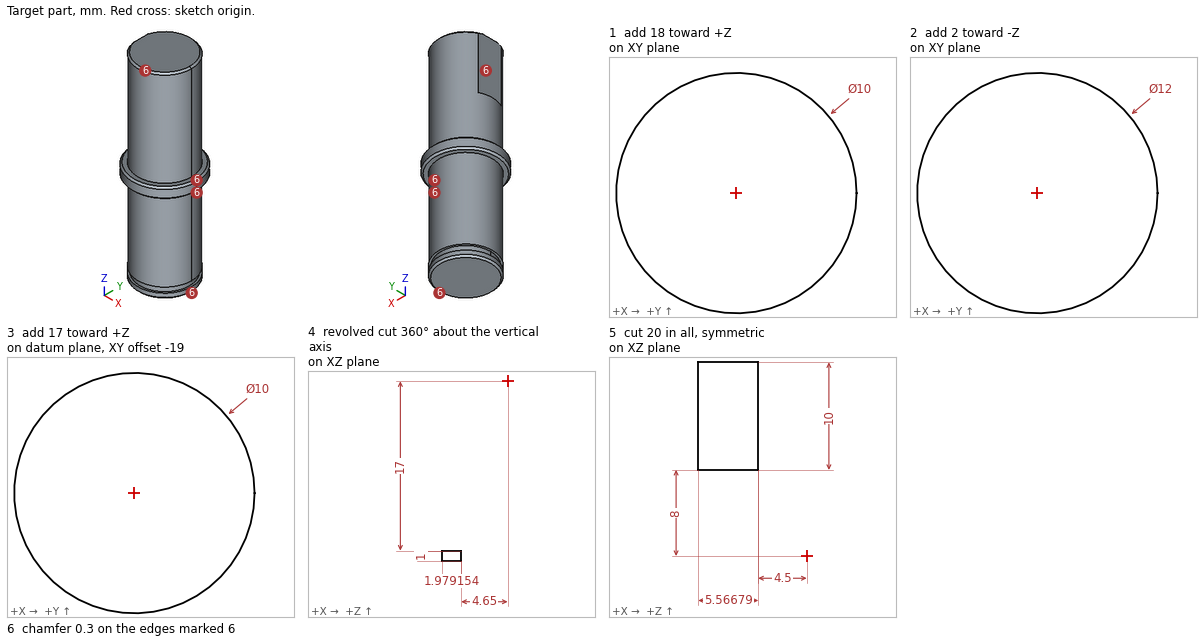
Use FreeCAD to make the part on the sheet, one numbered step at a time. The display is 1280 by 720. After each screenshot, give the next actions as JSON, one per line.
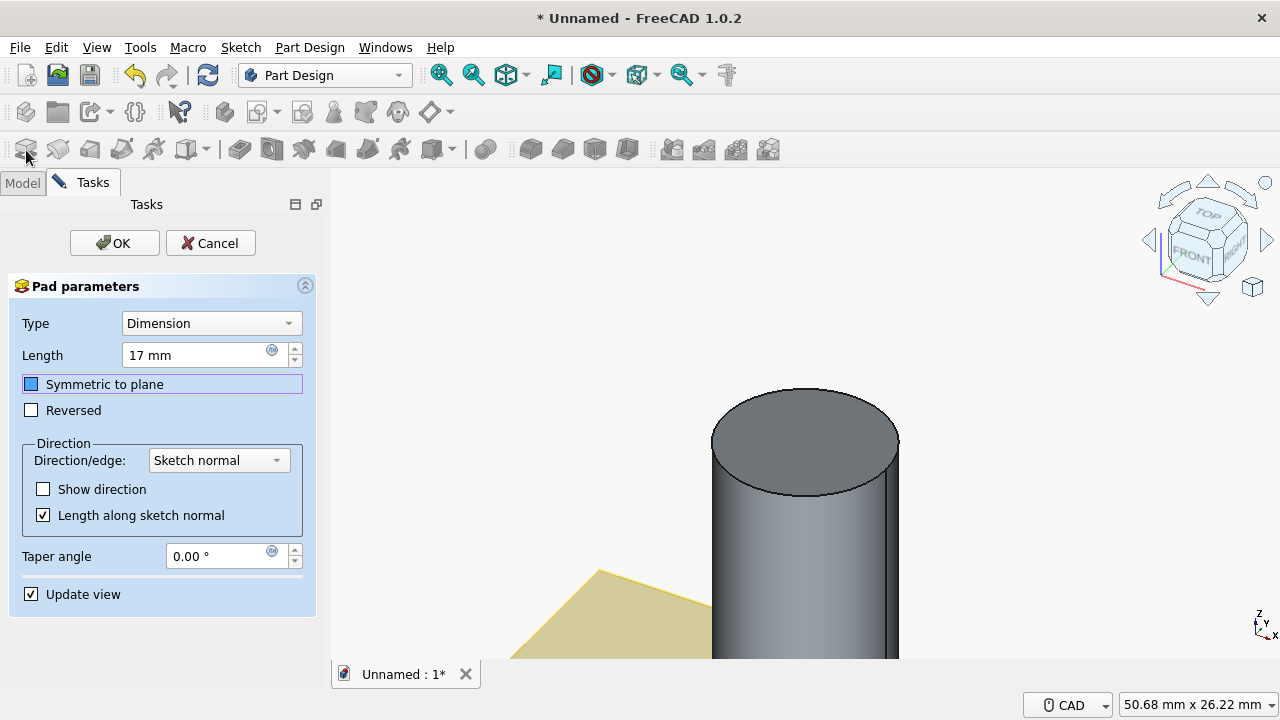
{"action": "left_click", "coordinate": [115, 243]}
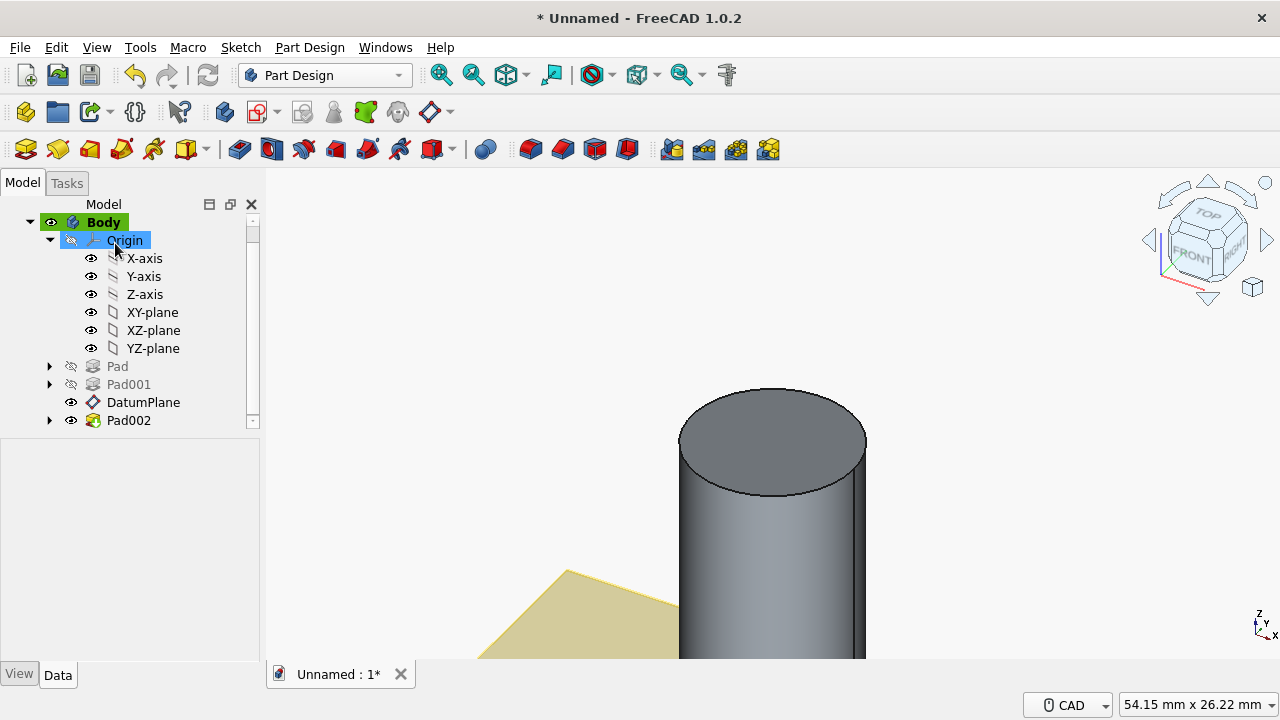
{"action": "left_click", "coordinate": [116, 402]}
{"action": "key", "text": "space"}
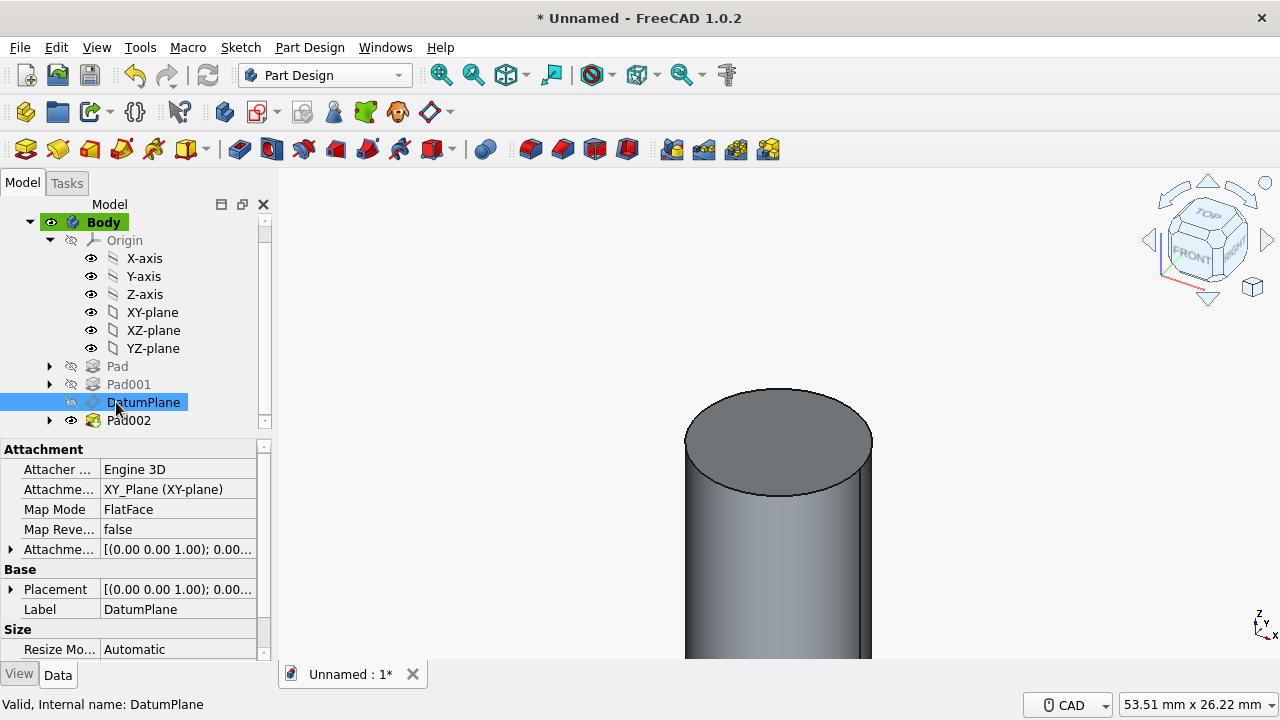
{"action": "left_click", "coordinate": [442, 76]}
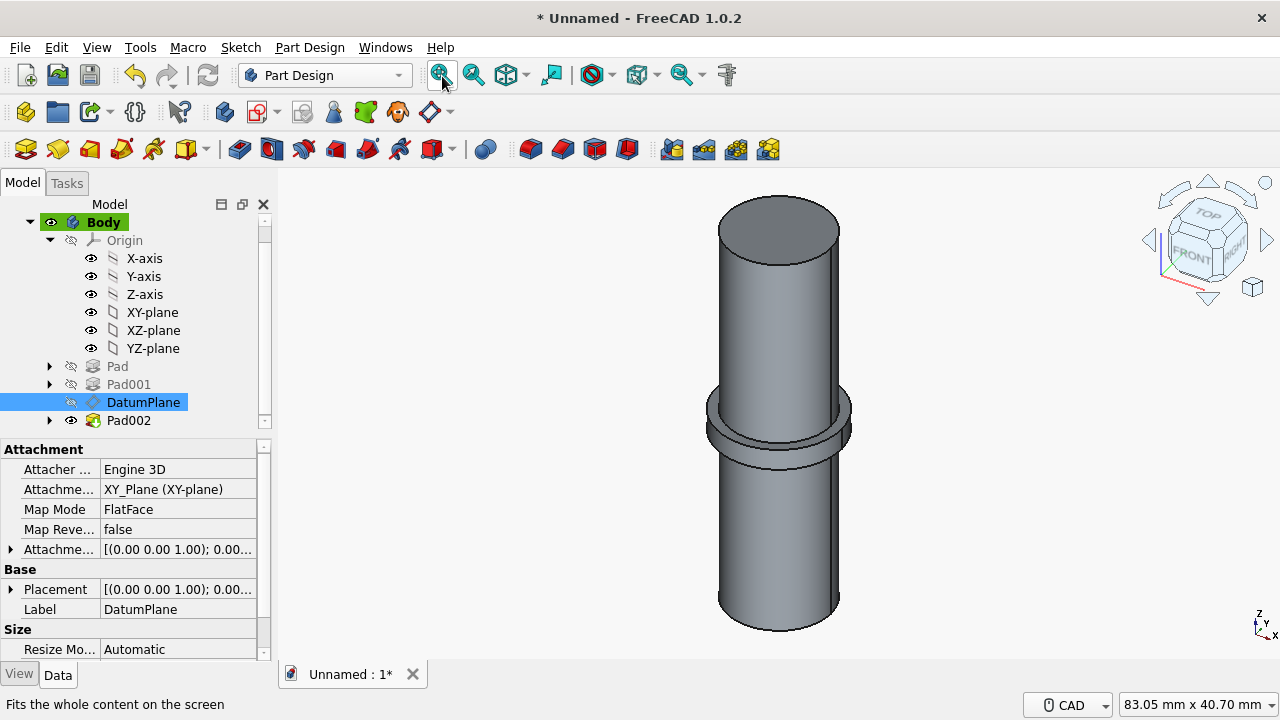
{"action": "left_click", "coordinate": [318, 619]}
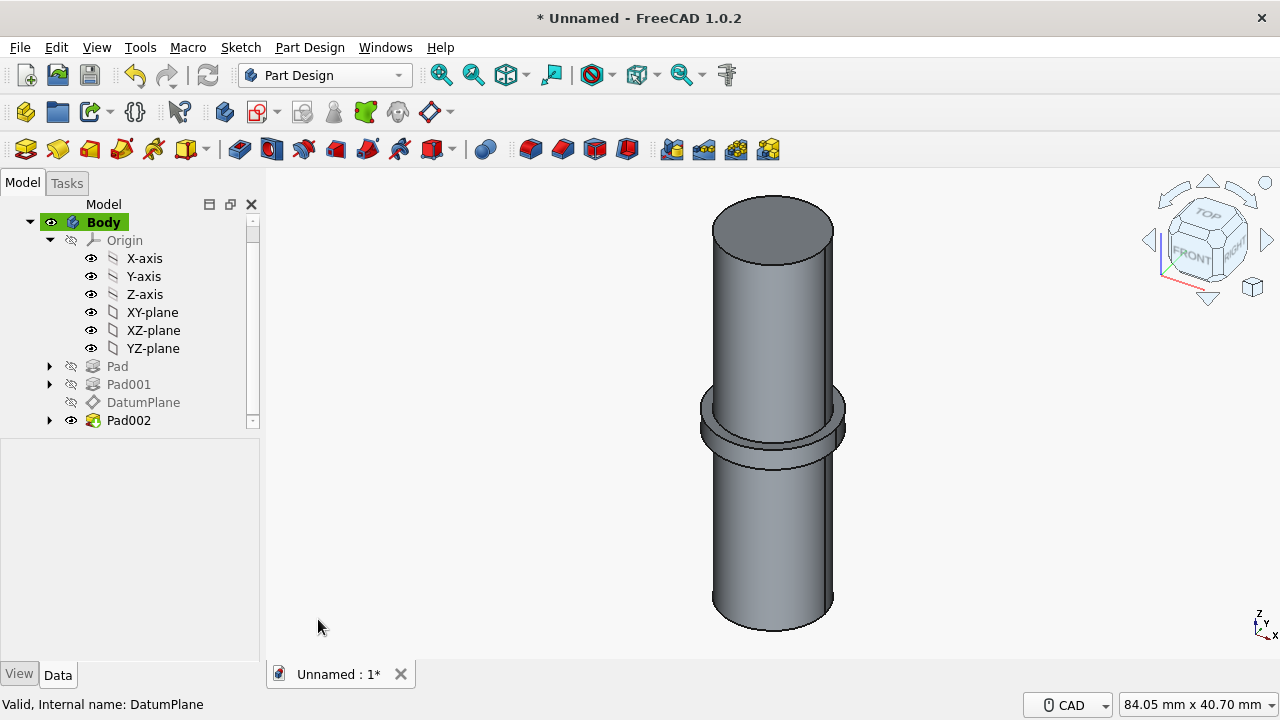
{"action": "left_click", "coordinate": [258, 112]}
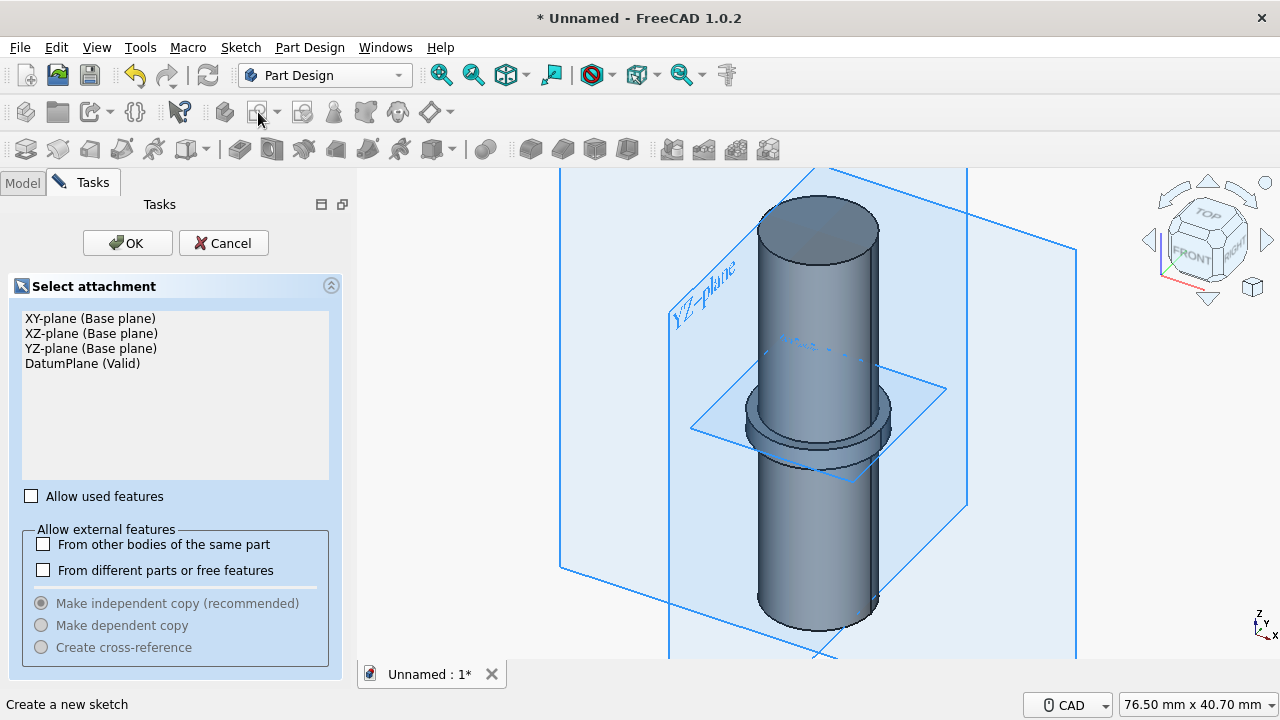
{"action": "left_click", "coordinate": [82, 334]}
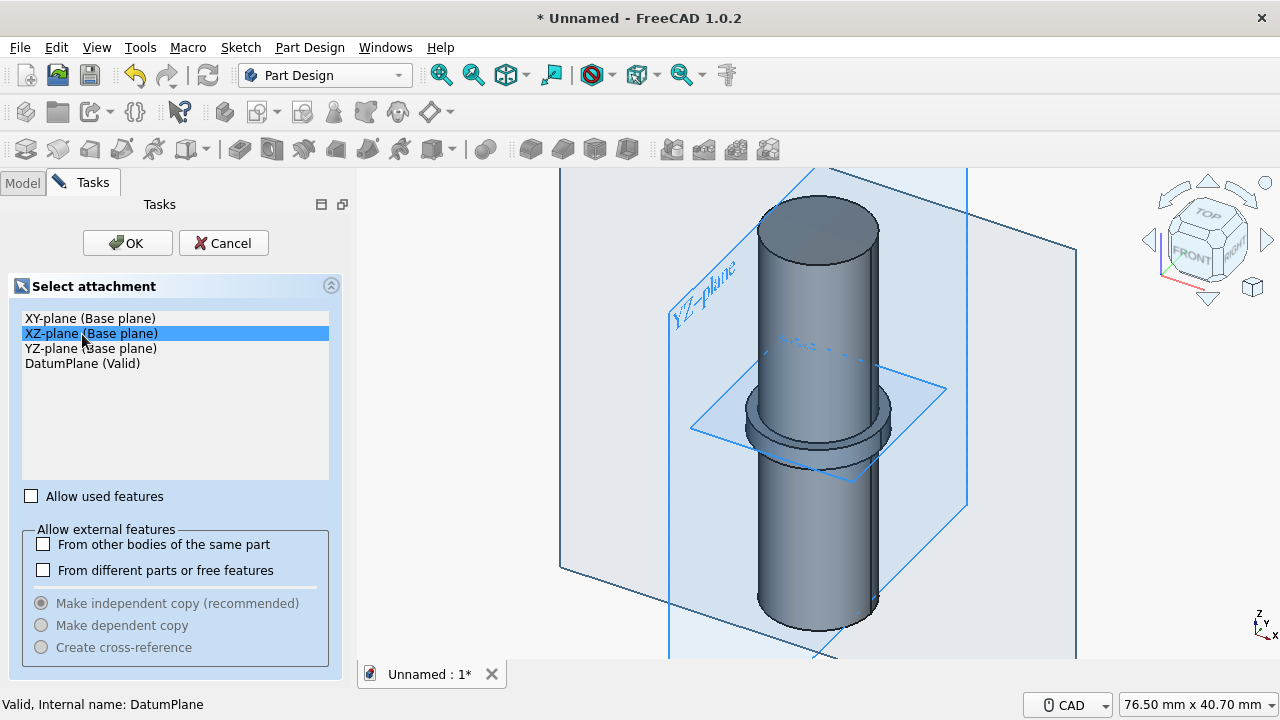
{"action": "left_click", "coordinate": [128, 243]}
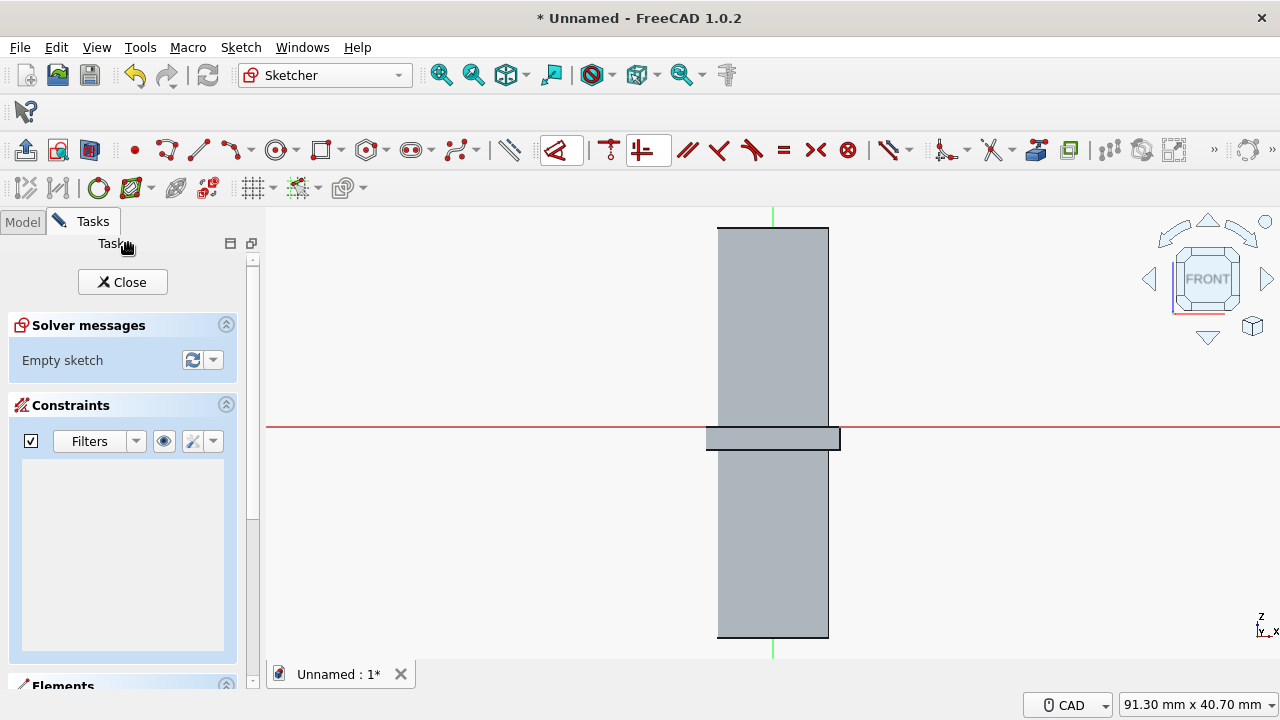
{"action": "left_click", "coordinate": [90, 150]}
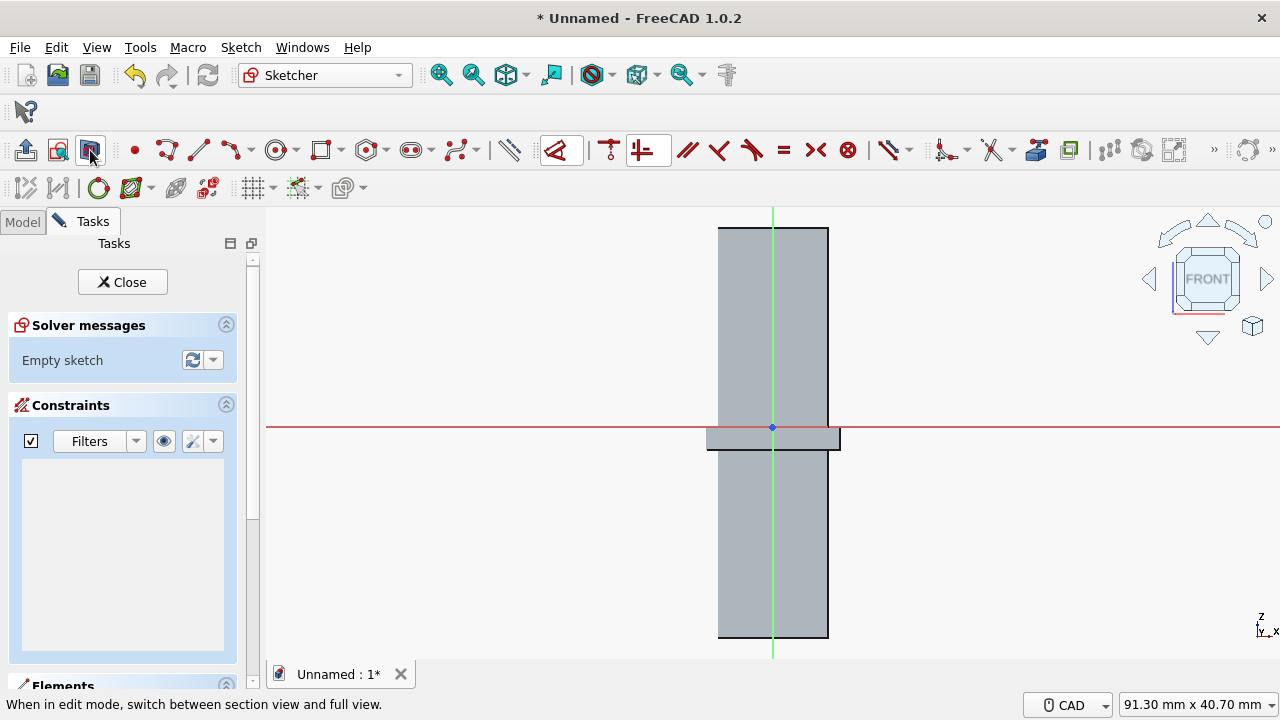
{"action": "scroll", "coordinate": [711, 631], "scroll_direction": "up", "scroll_amount": 15}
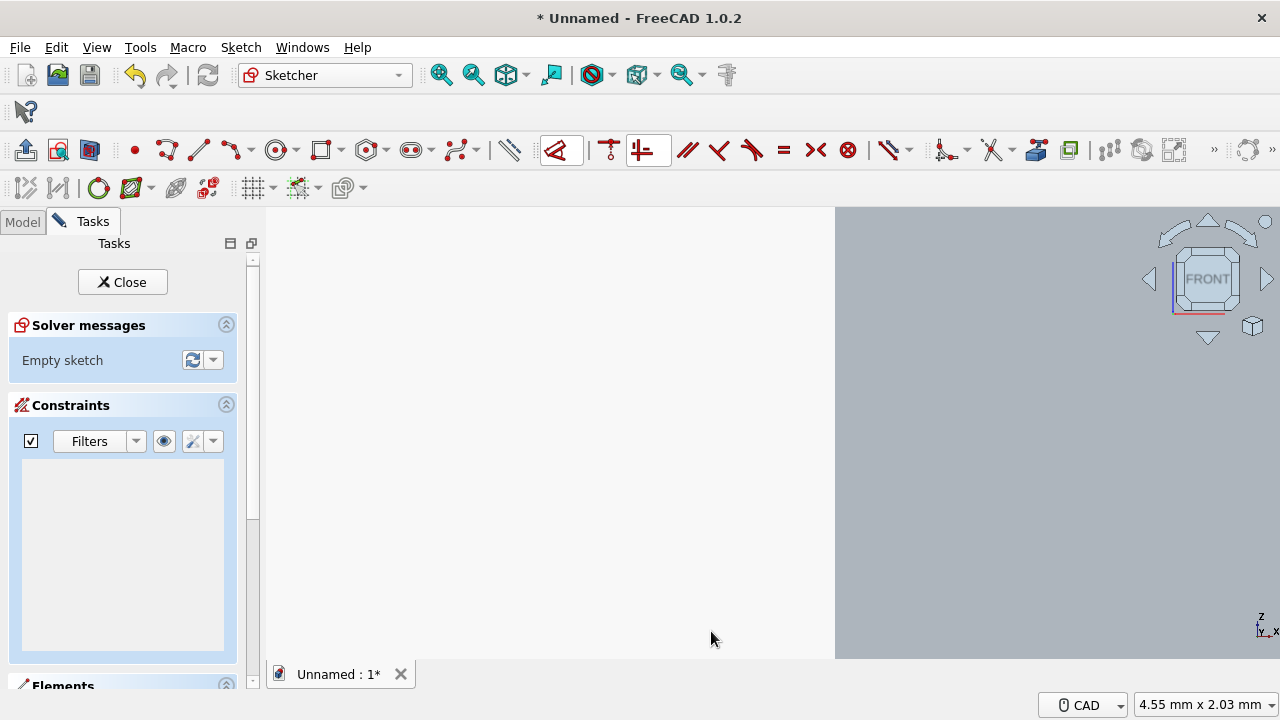
{"action": "left_click", "coordinate": [322, 150]}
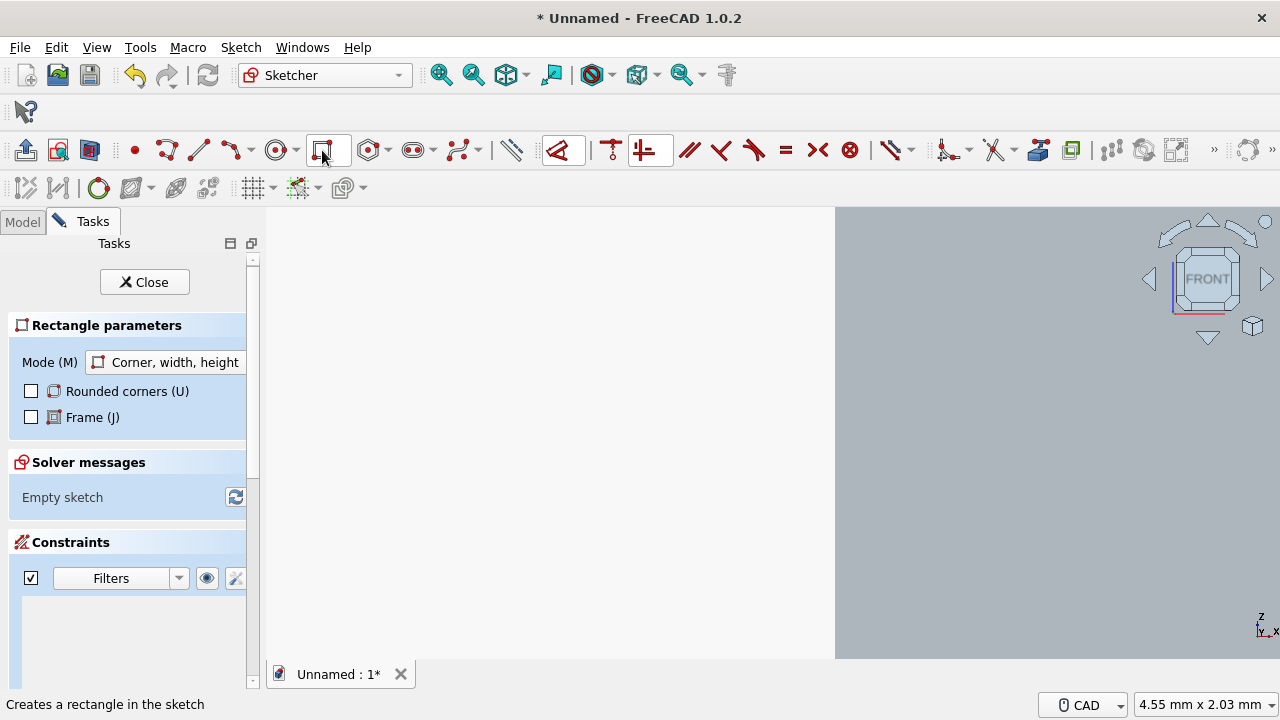
{"action": "left_click", "coordinate": [467, 317]}
{"action": "mouse_move", "coordinate": [908, 540]}